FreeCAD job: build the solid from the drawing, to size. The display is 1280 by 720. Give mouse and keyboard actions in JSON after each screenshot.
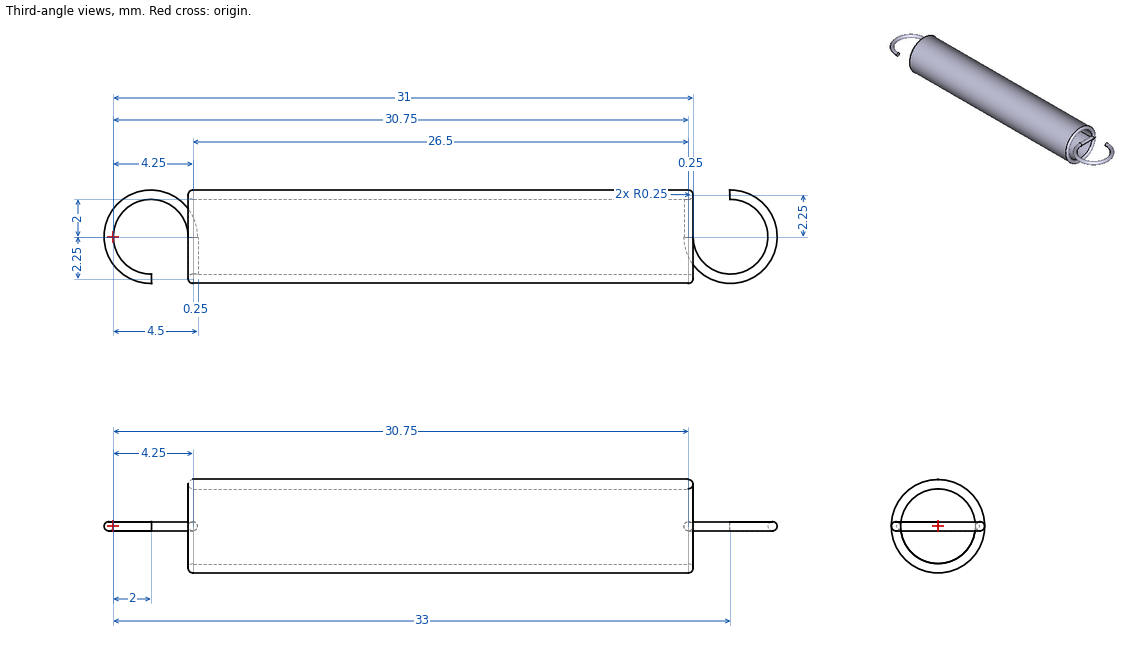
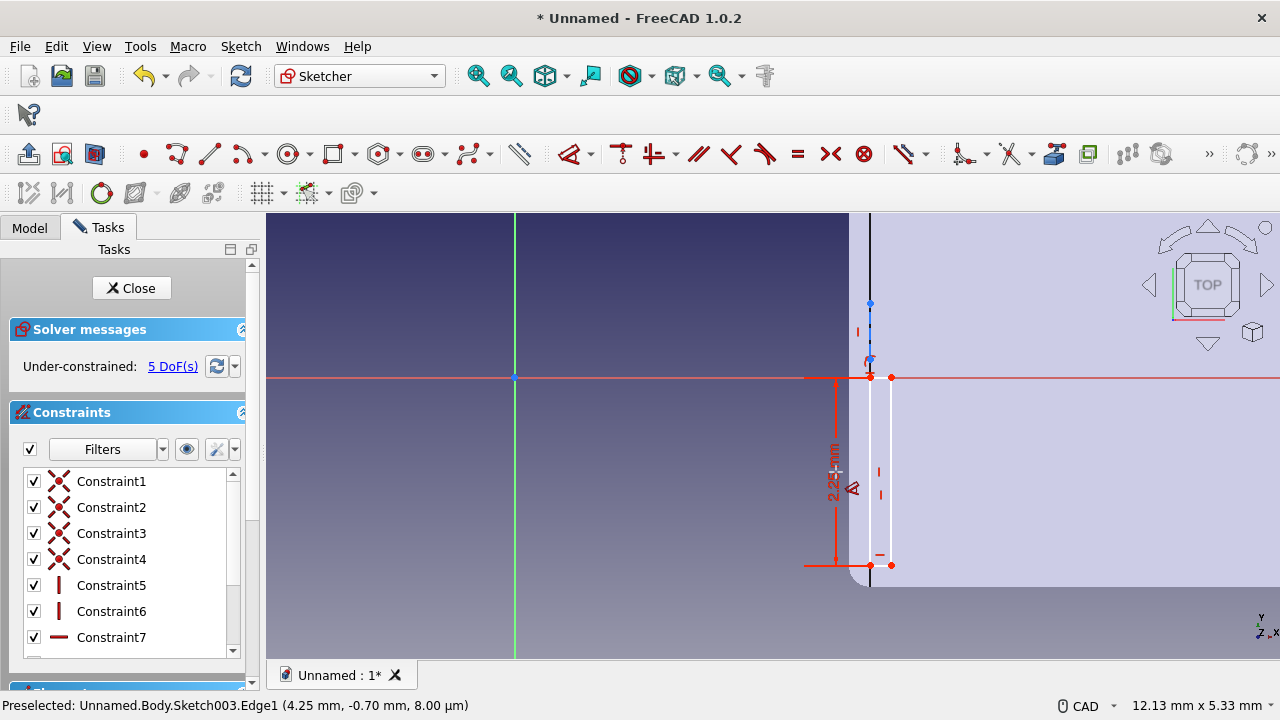
{"action": "scroll", "coordinate": [880, 566], "scroll_direction": "up", "scroll_amount": 4}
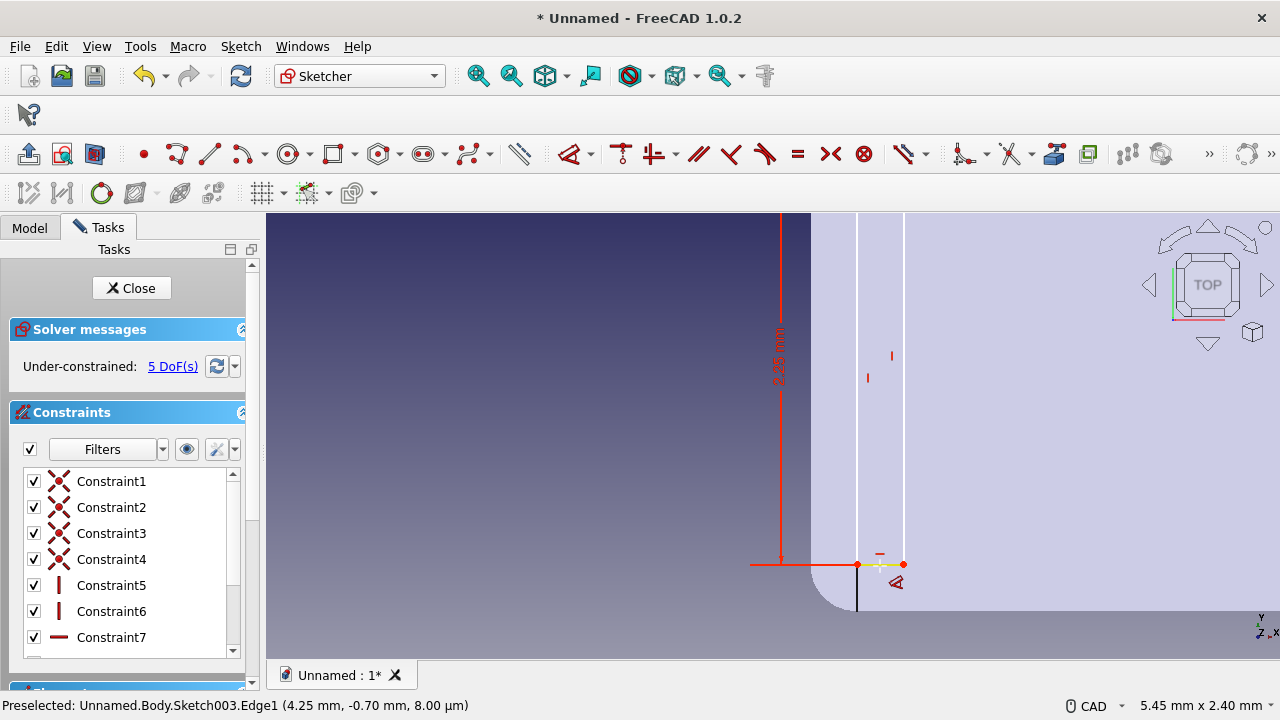
{"action": "left_click", "coordinate": [880, 565]}
{"action": "left_click", "coordinate": [880, 599]}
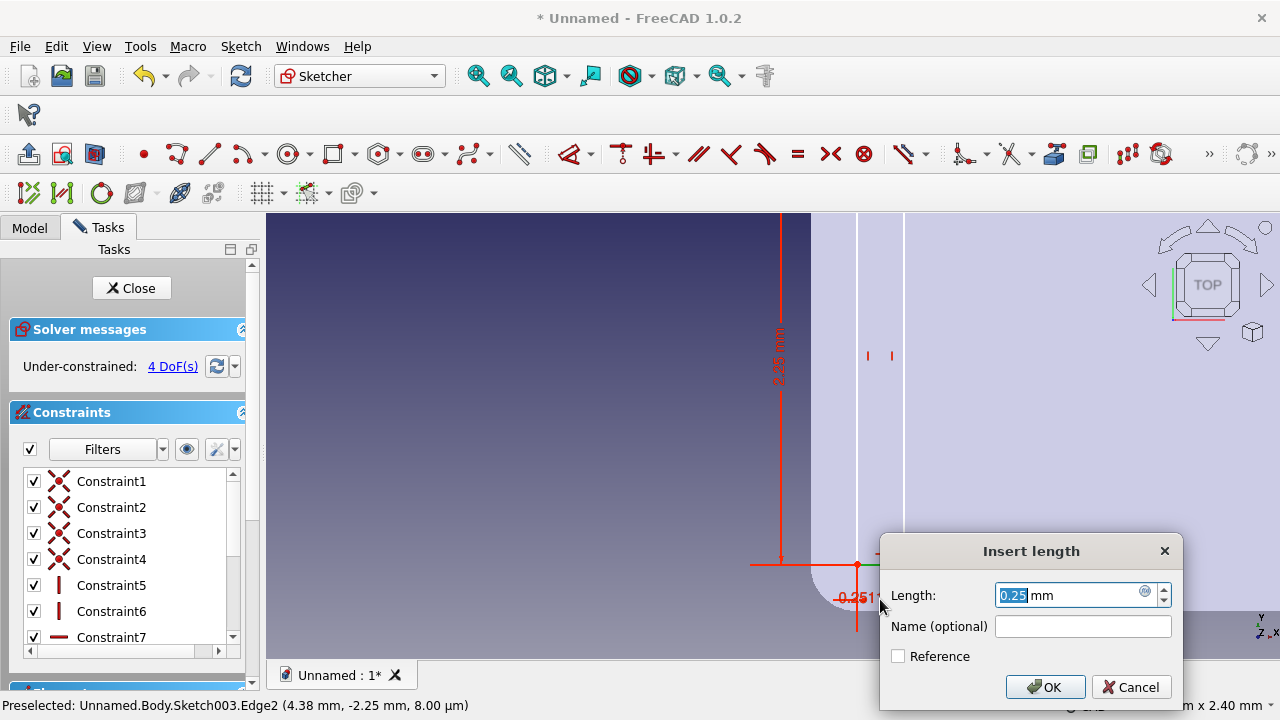
{"action": "type", "text": "0.25"}
{"action": "key", "text": "Return"}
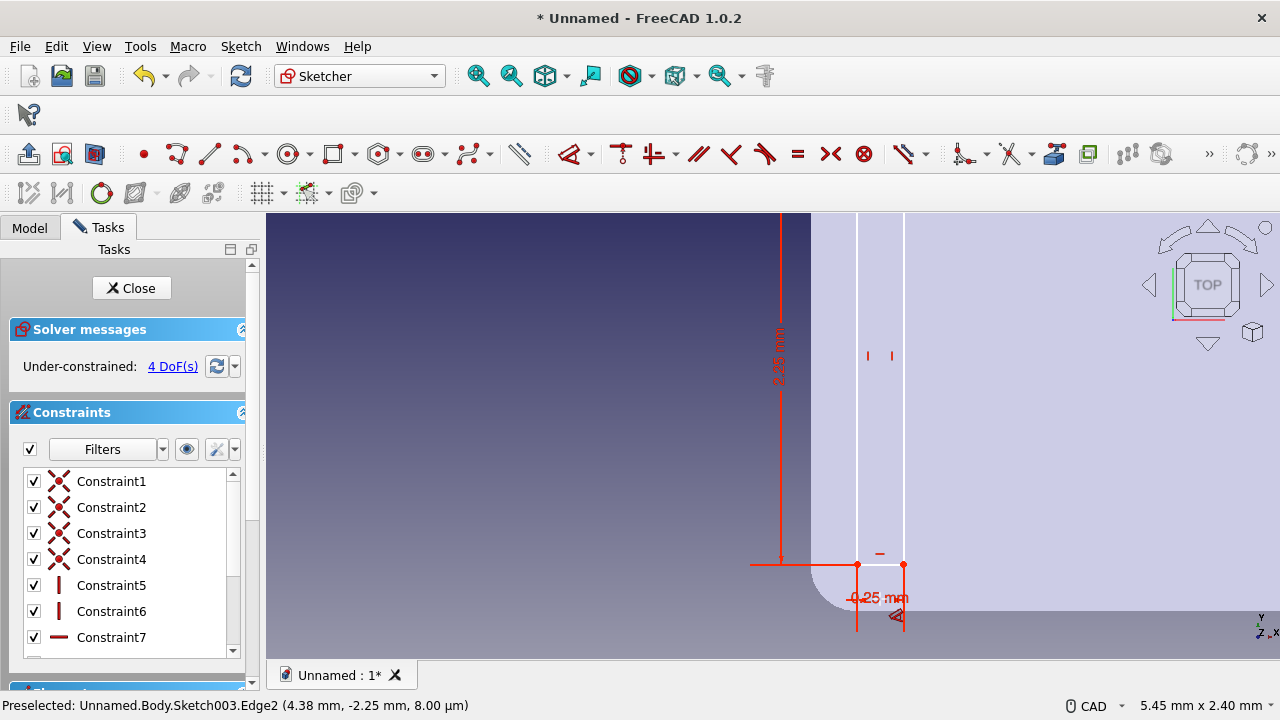
{"action": "left_click", "coordinate": [904, 565]}
{"action": "left_click", "coordinate": [599, 599]}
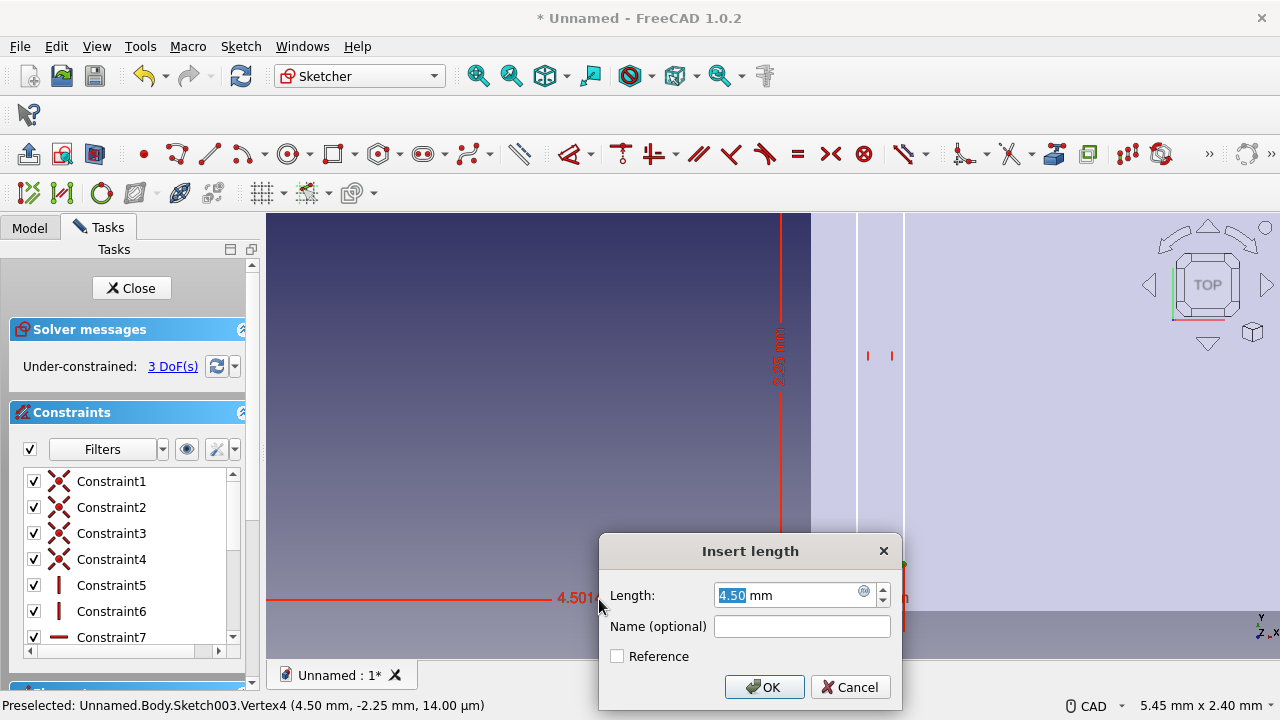
{"action": "type", "text": "4.5"}
{"action": "key", "text": "Return"}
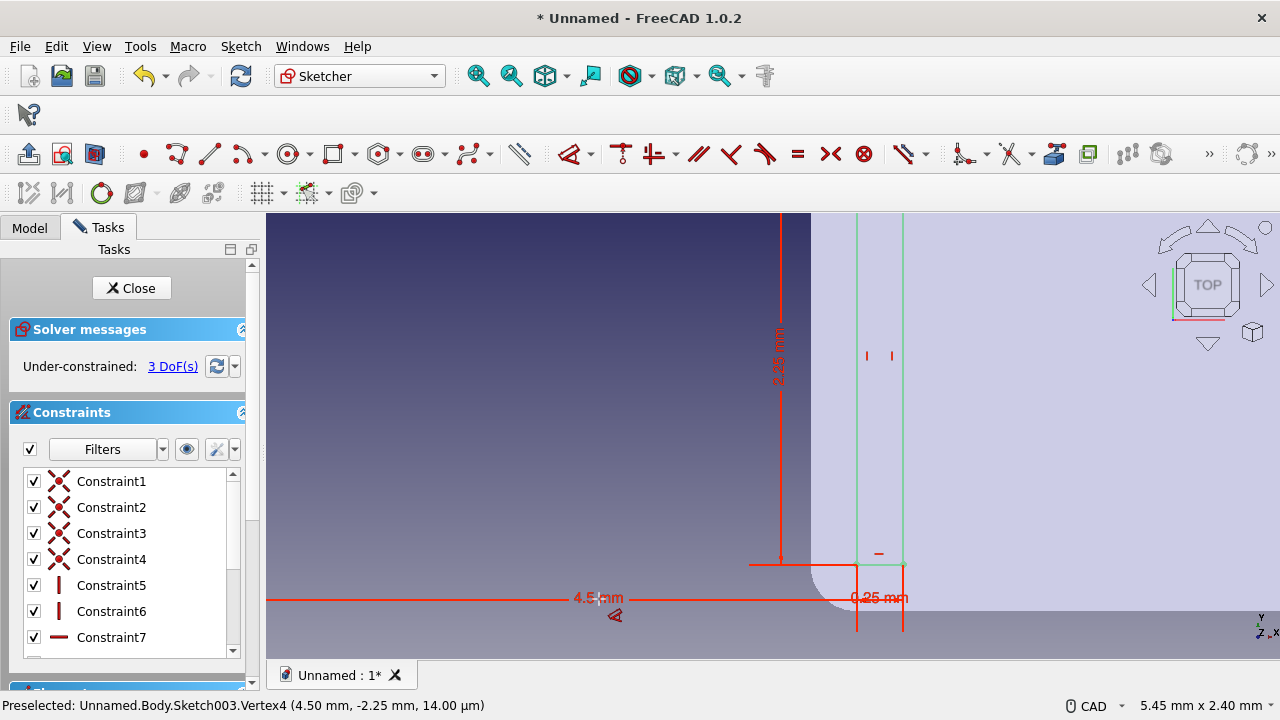
{"action": "scroll", "coordinate": [884, 570], "scroll_direction": "down", "scroll_amount": 4}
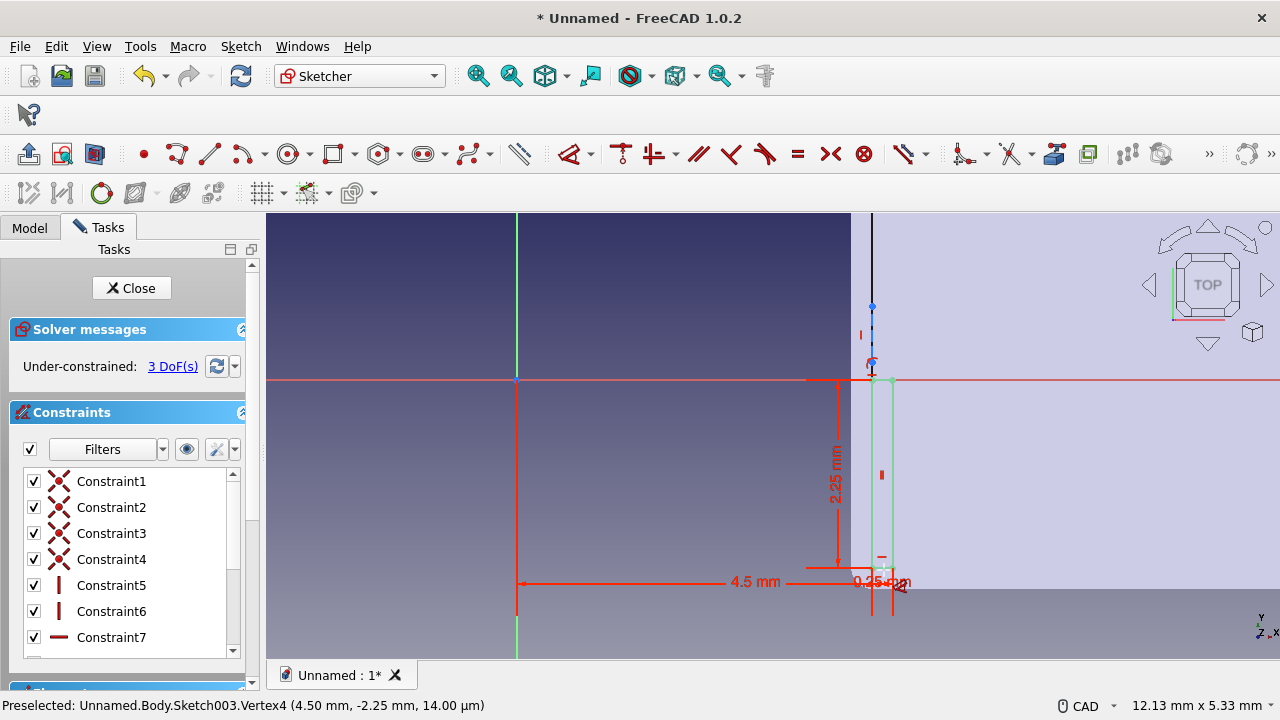
{"action": "left_click", "coordinate": [872, 362]}
{"action": "left_click", "coordinate": [694, 328]}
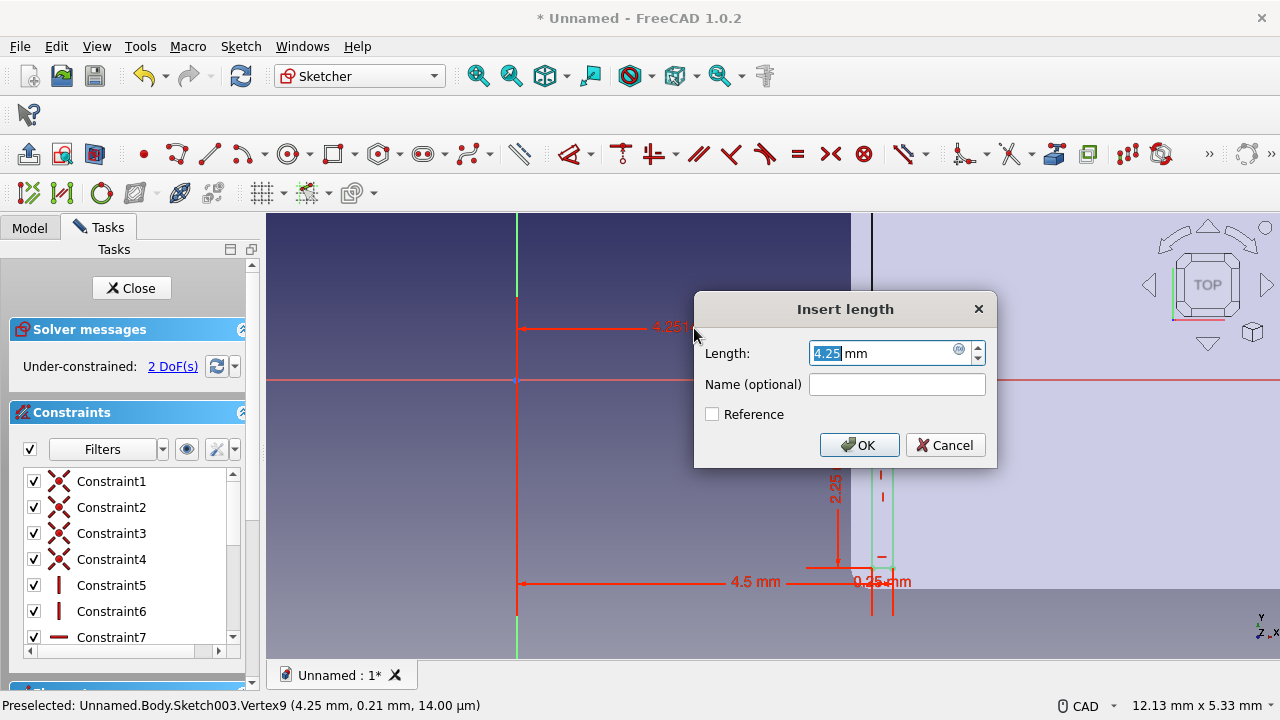
{"action": "type", "text": "4.25"}
{"action": "key", "text": "Return"}
{"action": "key", "text": "Escape"}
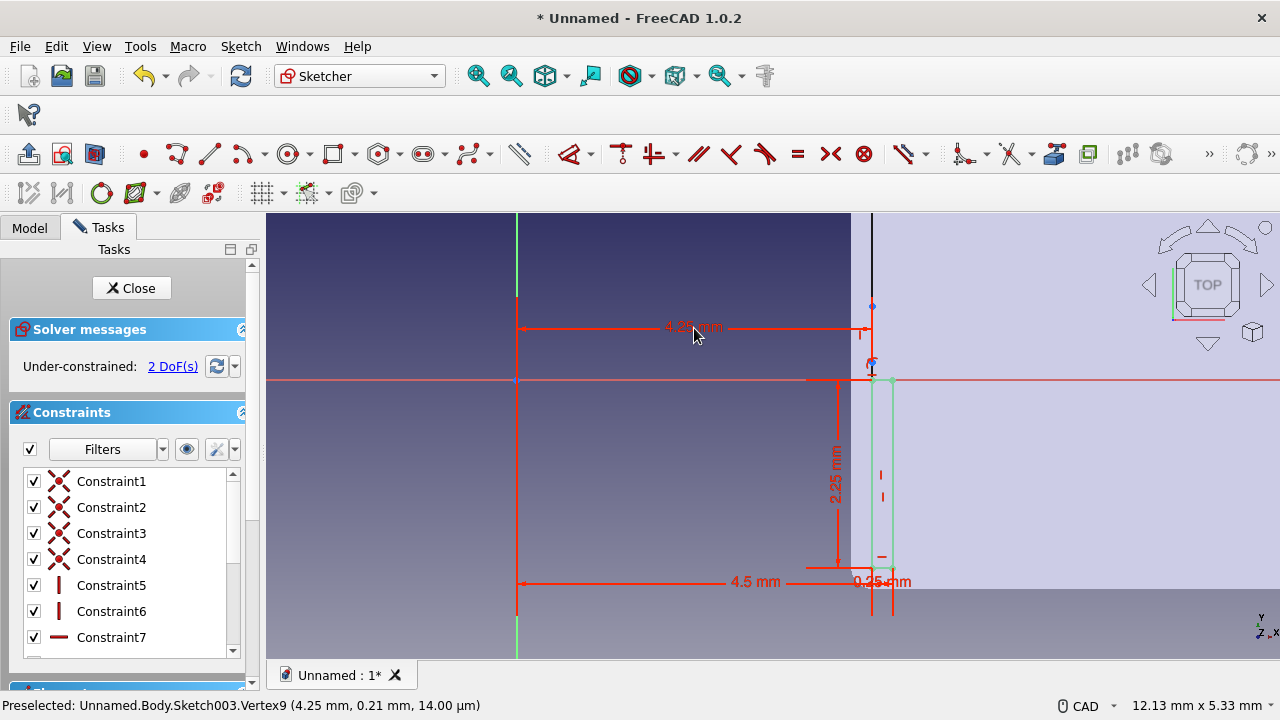
{"action": "left_click", "coordinate": [132, 288]}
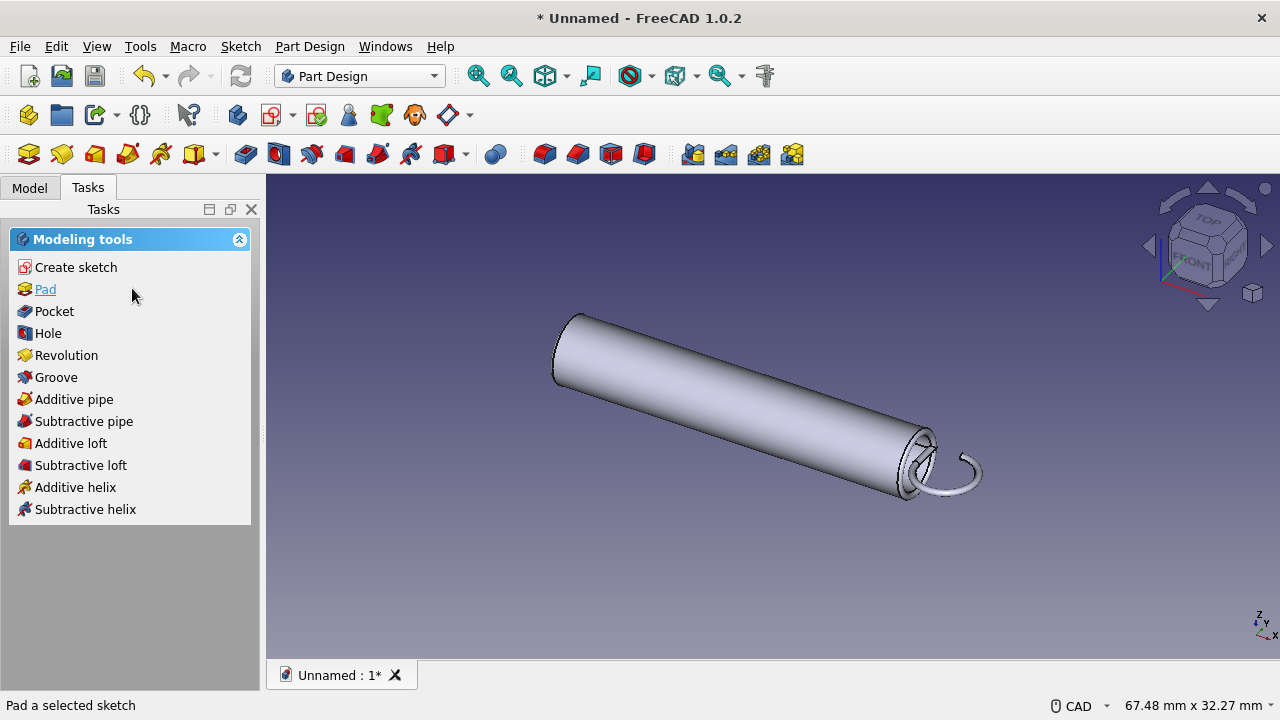
{"action": "left_click", "coordinate": [62, 154]}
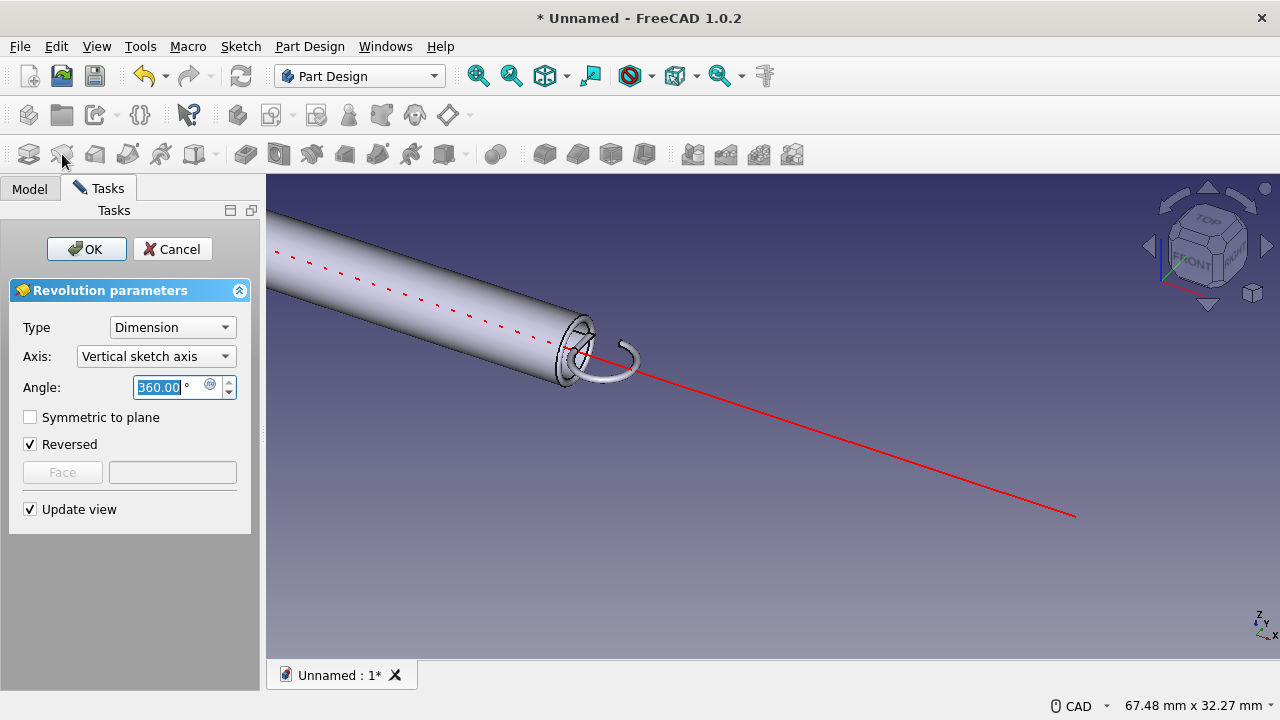
{"action": "left_click", "coordinate": [157, 356]}